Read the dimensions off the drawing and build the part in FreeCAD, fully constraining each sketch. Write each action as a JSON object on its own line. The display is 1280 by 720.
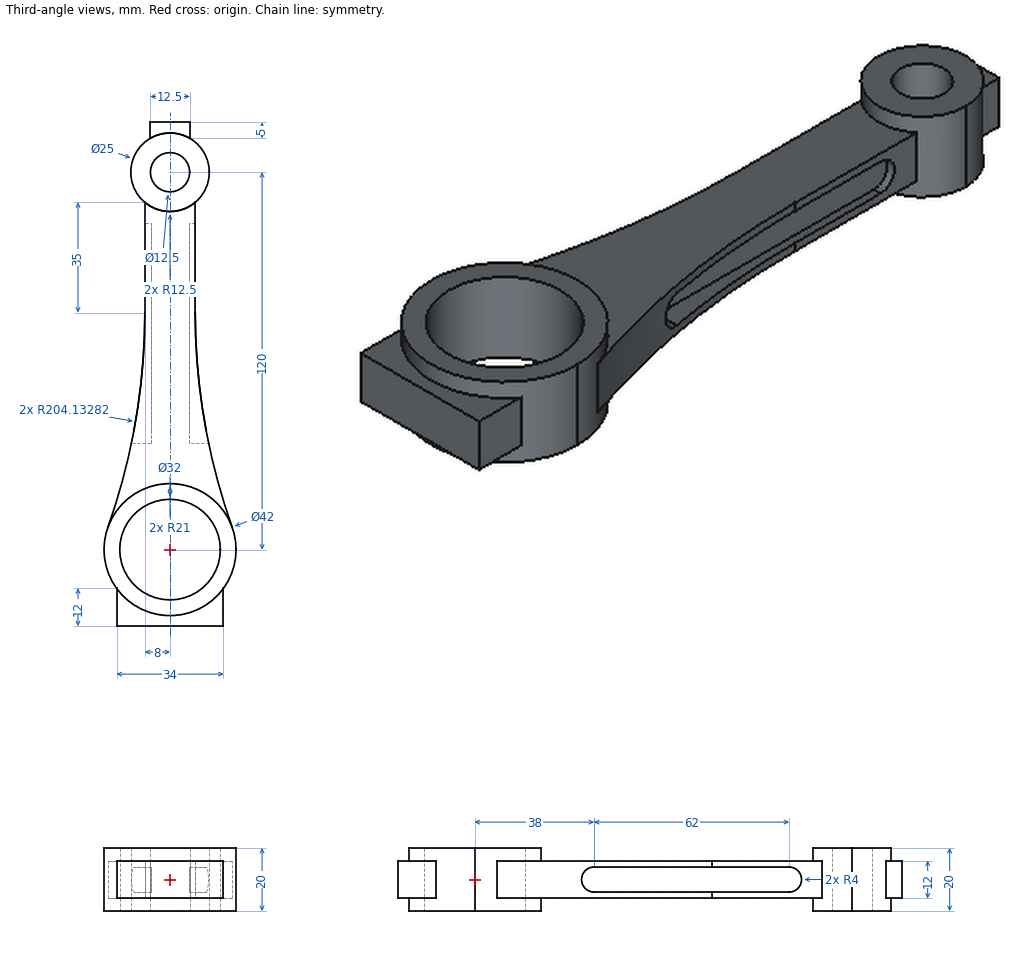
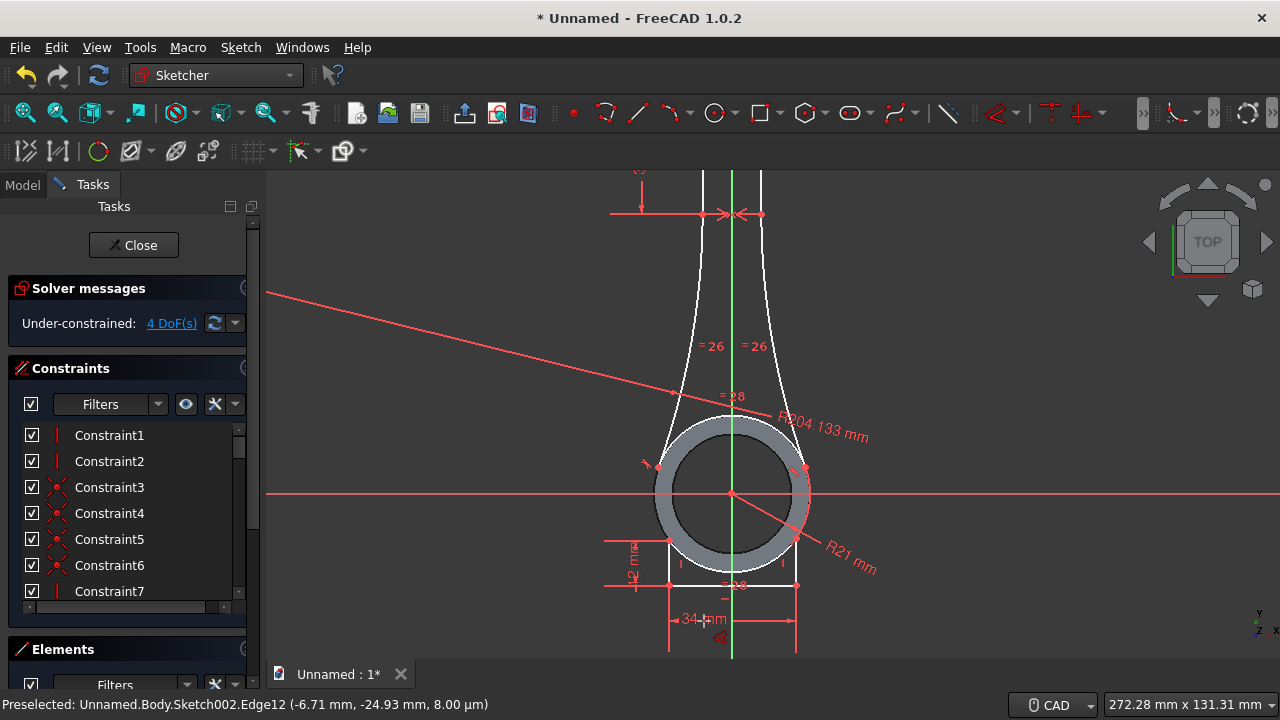
{"action": "left_click", "coordinate": [796, 572]}
{"action": "left_click", "coordinate": [762, 551]}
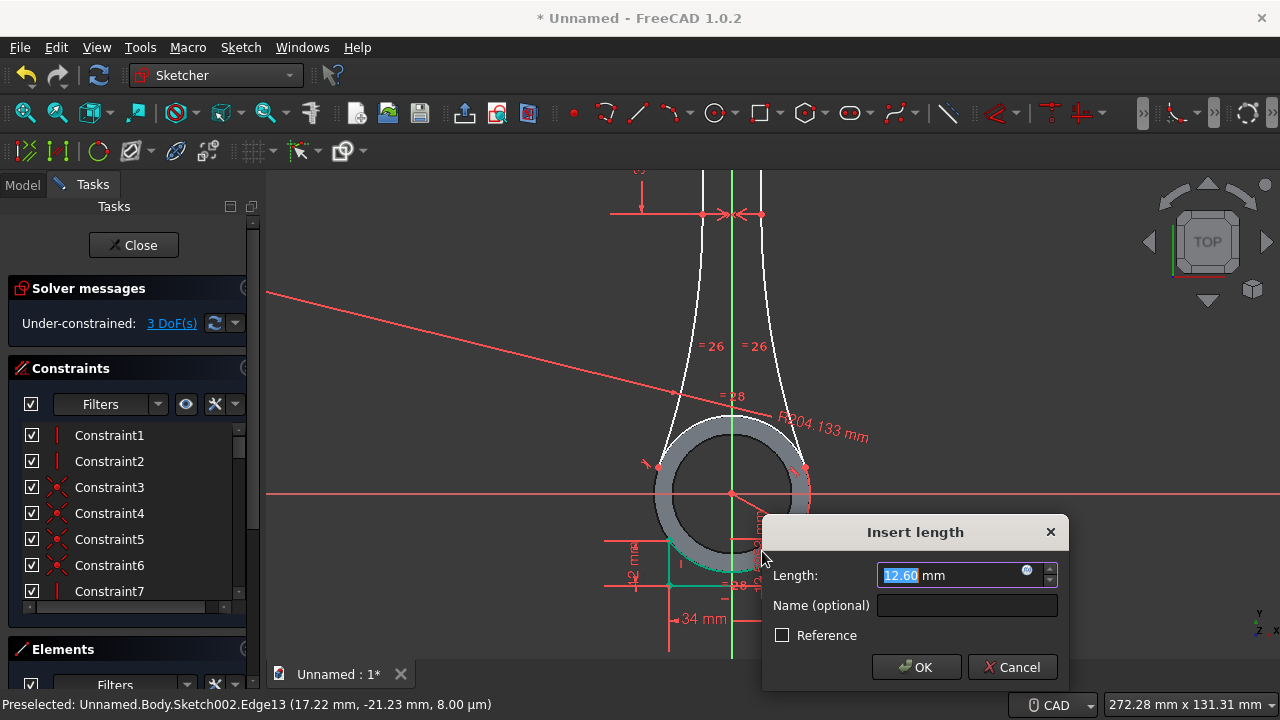
{"action": "type", "text": "12"}
{"action": "key", "text": "Return"}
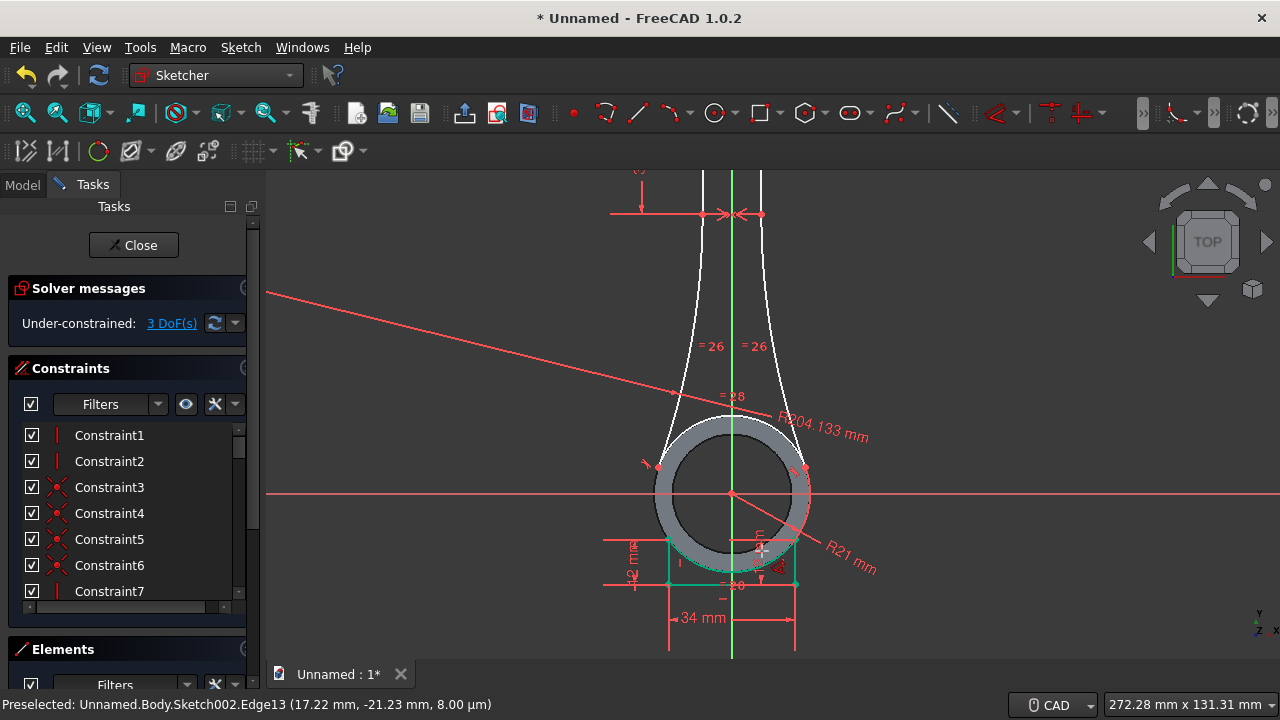
{"action": "scroll", "coordinate": [671, 570], "scroll_direction": "down", "scroll_amount": 3}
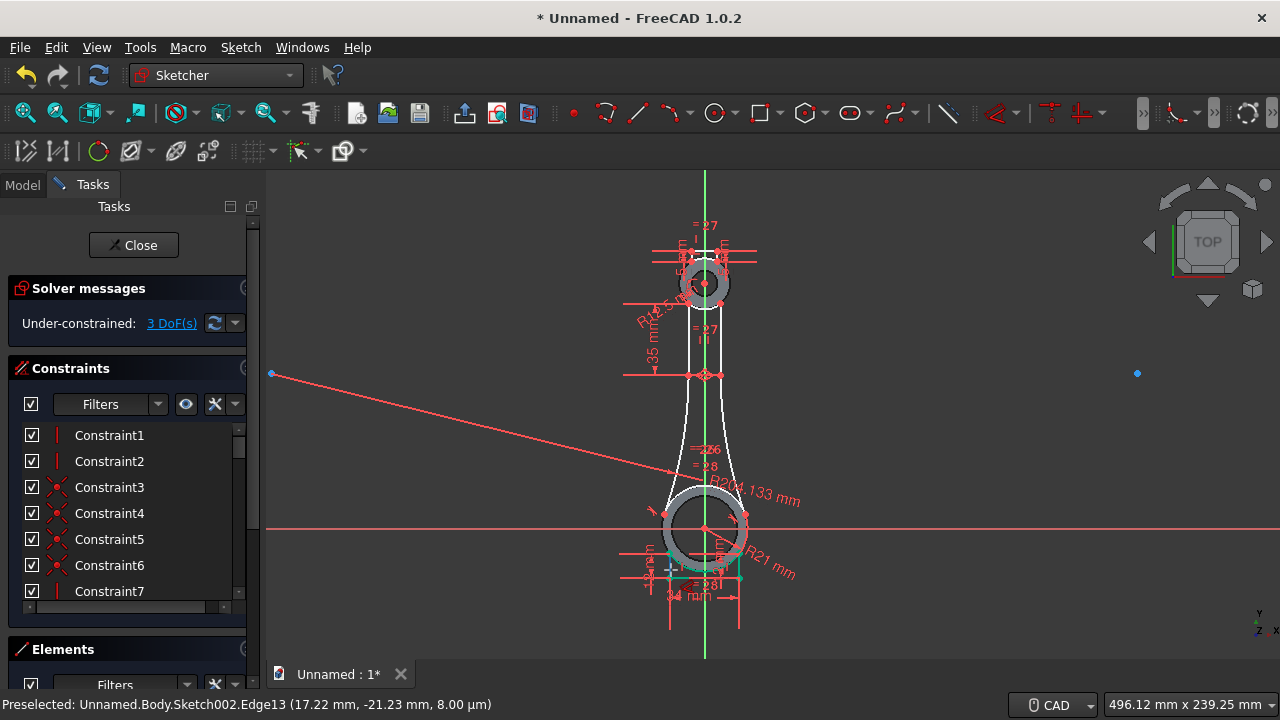
{"action": "scroll", "coordinate": [689, 304], "scroll_direction": "up", "scroll_amount": 5}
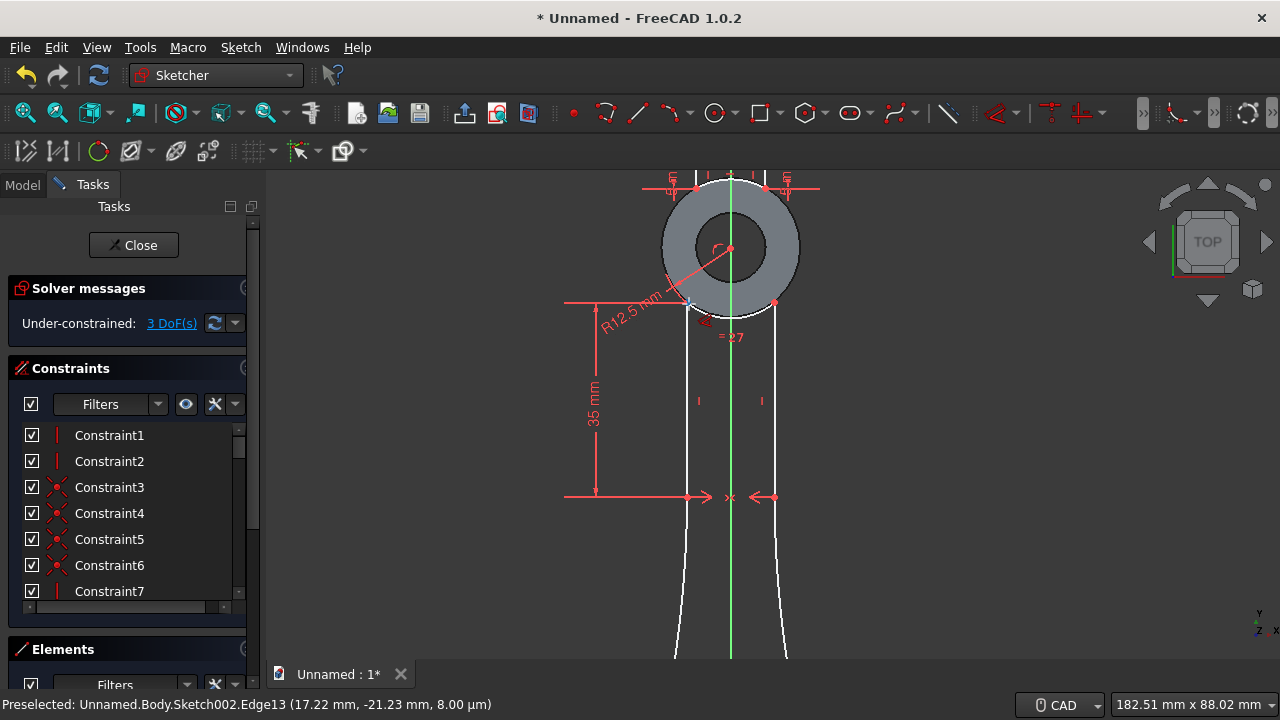
{"action": "left_click", "coordinate": [687, 303]}
{"action": "left_click", "coordinate": [709, 269]}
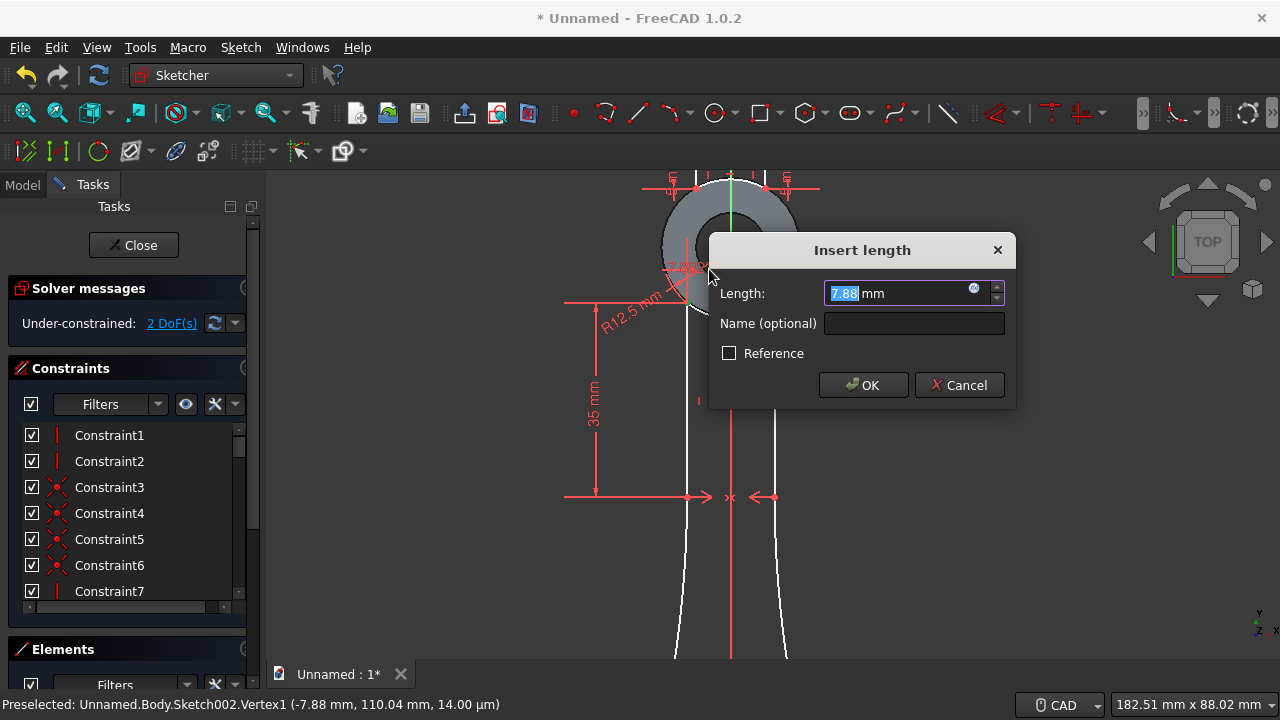
{"action": "type", "text": "8"}
{"action": "key", "text": "Return"}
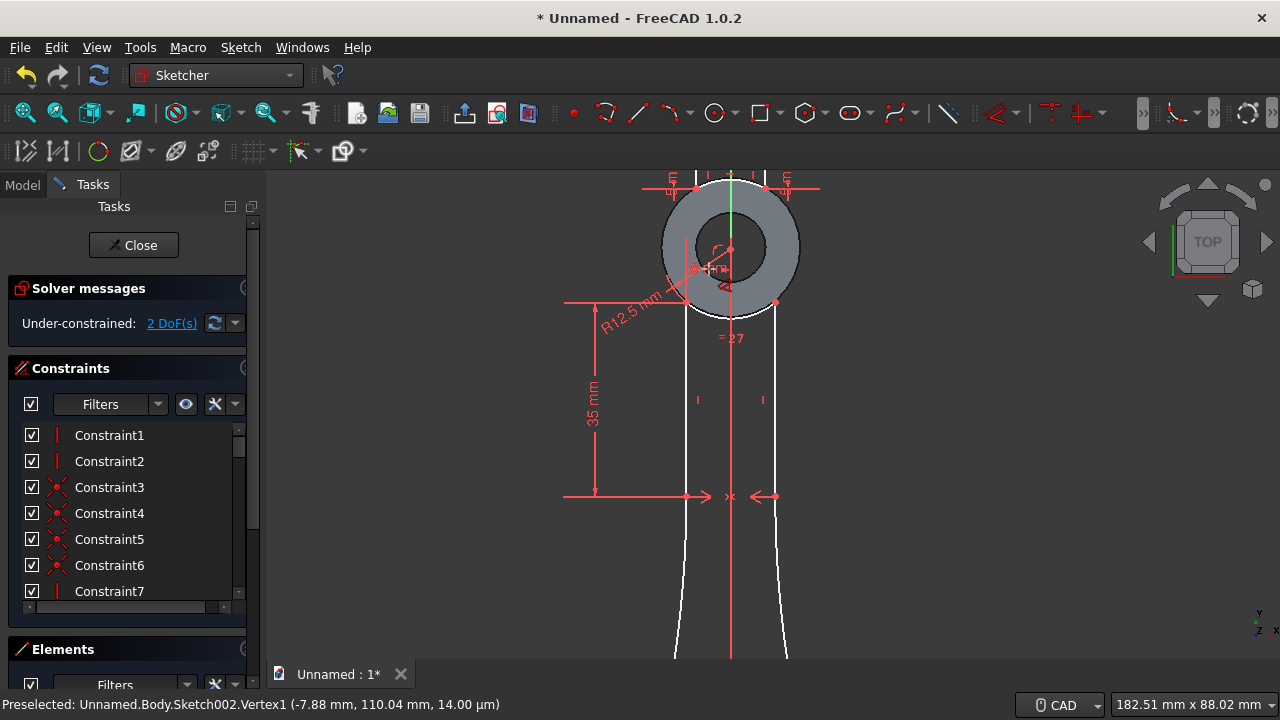
{"action": "scroll", "coordinate": [689, 304], "scroll_direction": "down", "scroll_amount": 5}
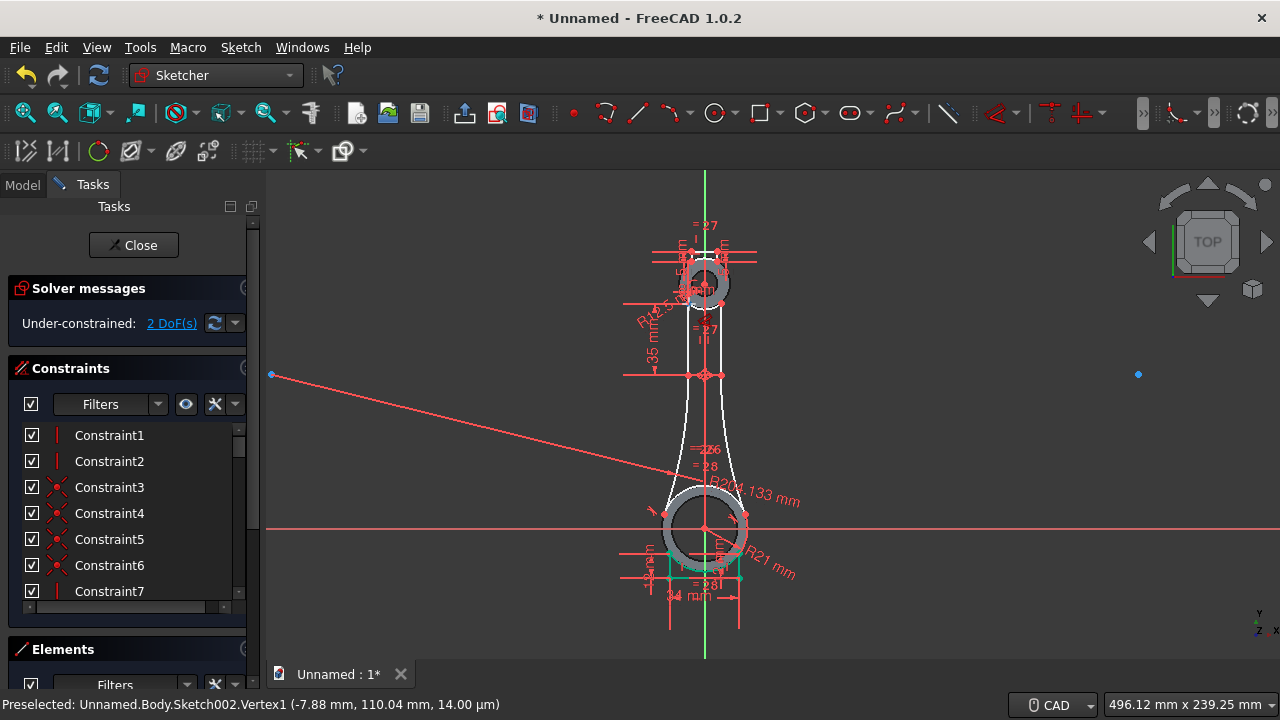
{"action": "scroll", "coordinate": [710, 252], "scroll_direction": "up", "scroll_amount": 6}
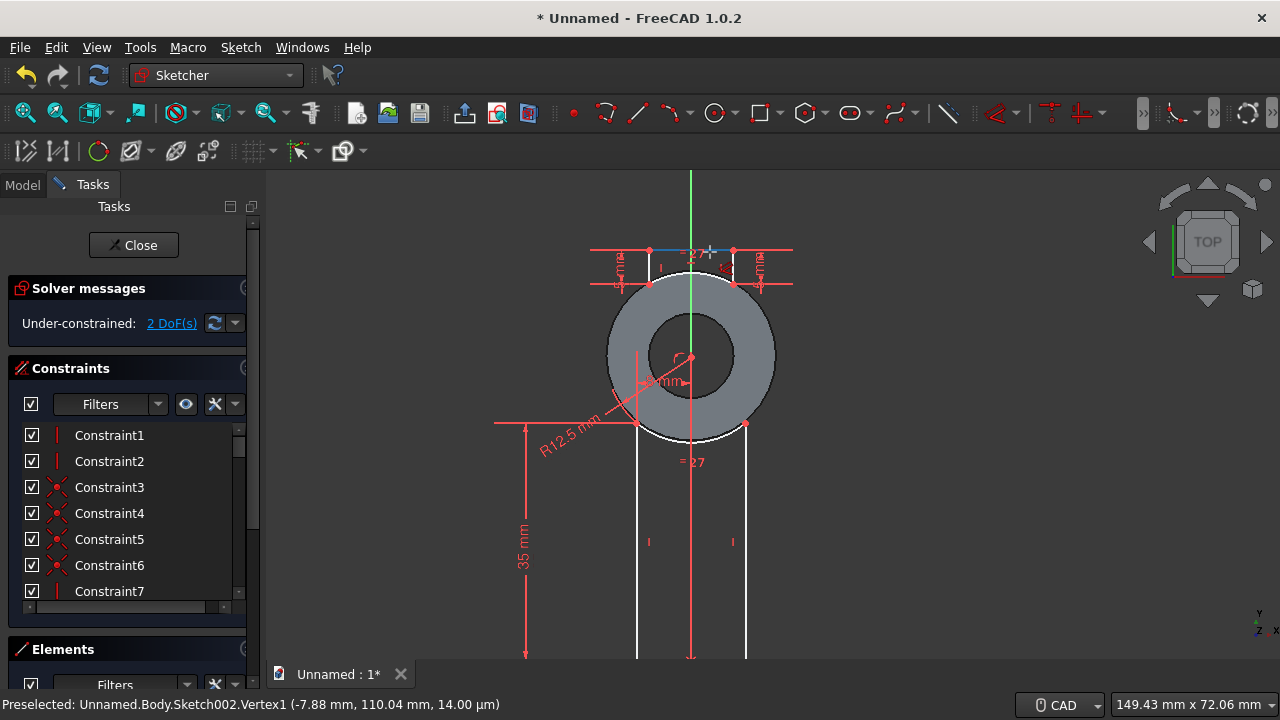
{"action": "left_click", "coordinate": [708, 250]}
{"action": "left_click", "coordinate": [672, 216]}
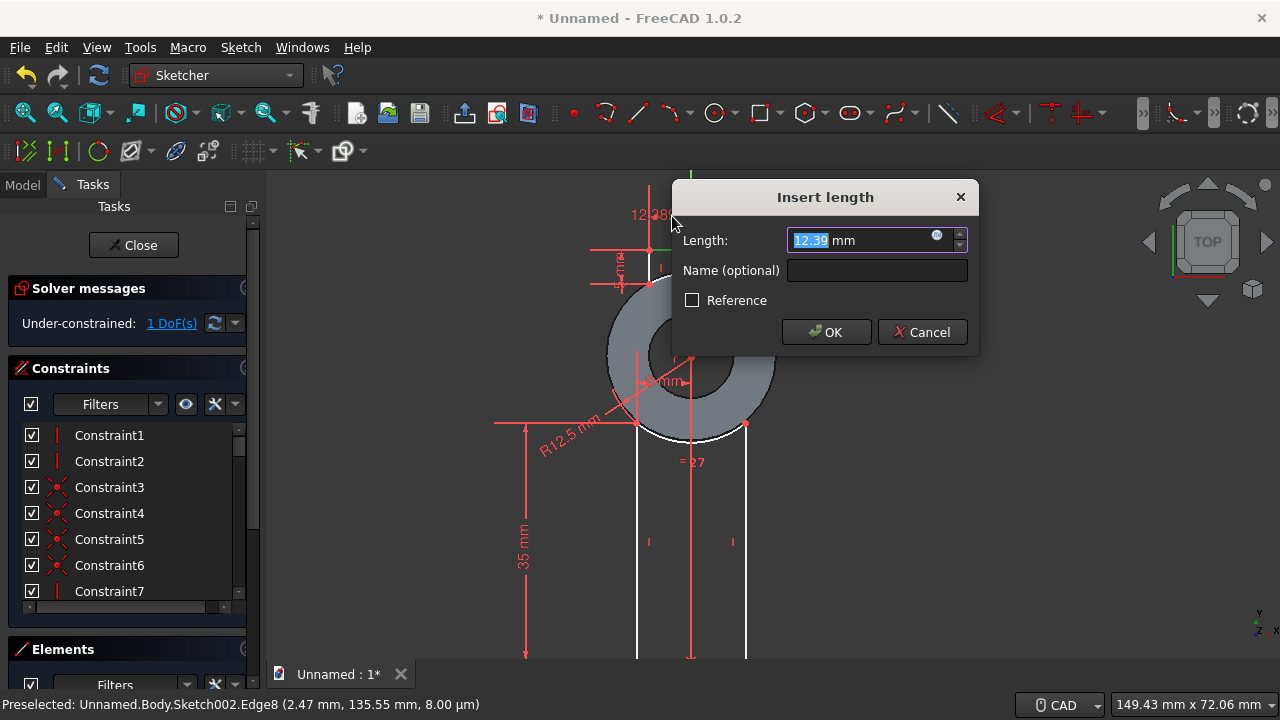
{"action": "type", "text": "12.5"}
{"action": "key", "text": "Return"}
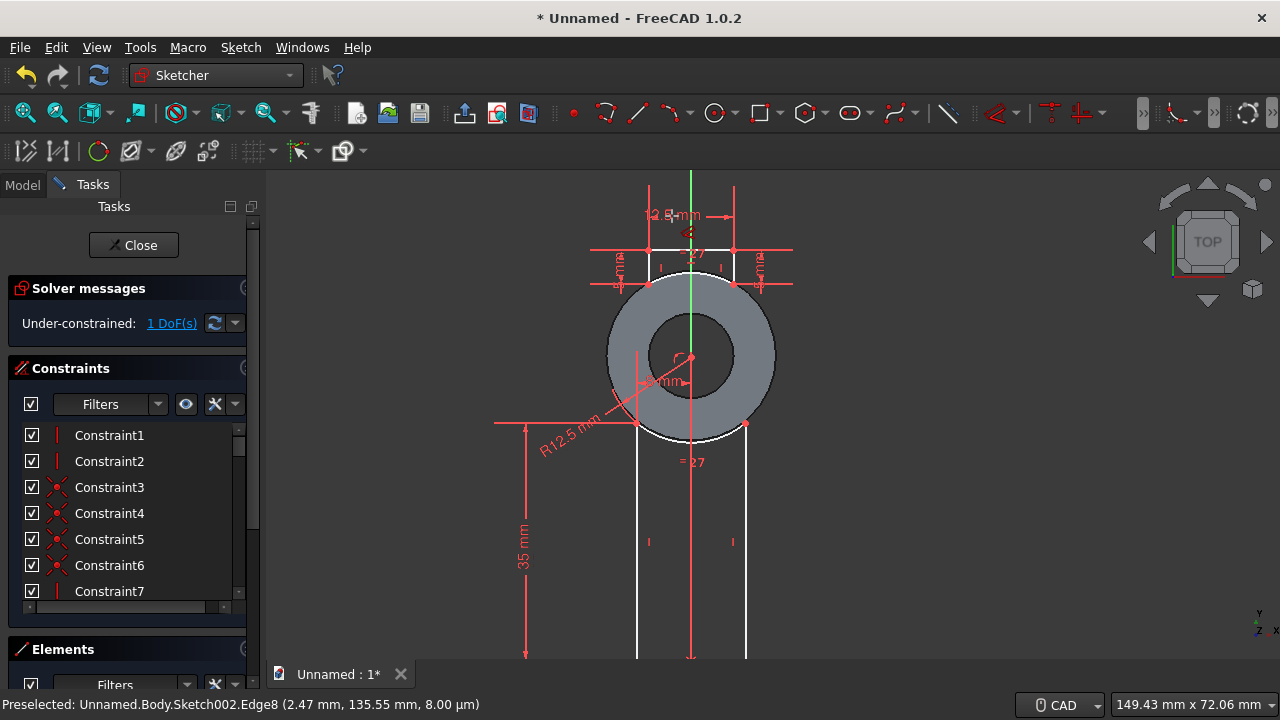
{"action": "left_click", "coordinate": [691, 358]}
{"action": "left_click", "coordinate": [725, 494]}